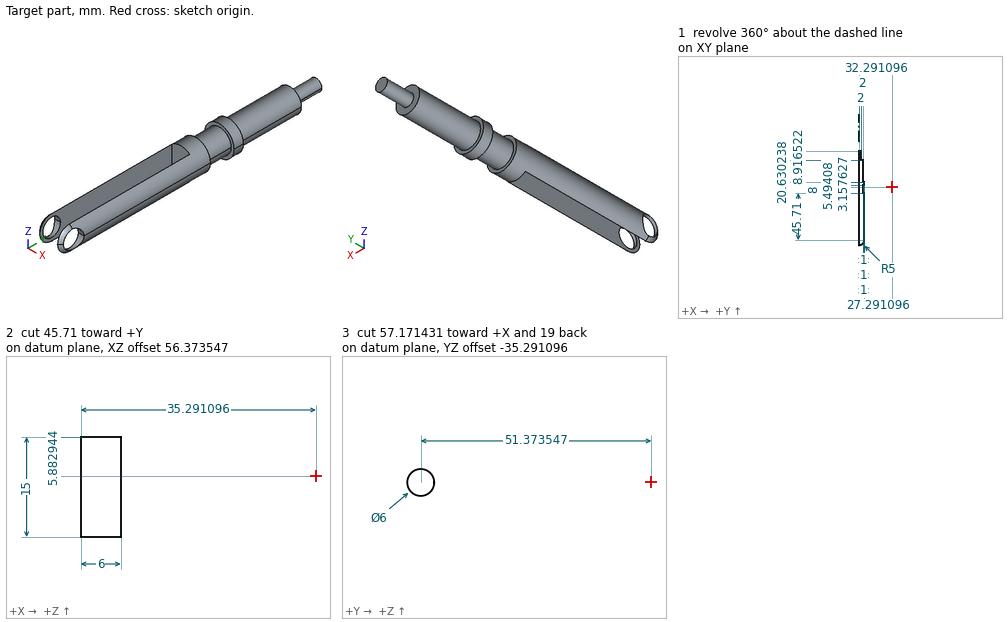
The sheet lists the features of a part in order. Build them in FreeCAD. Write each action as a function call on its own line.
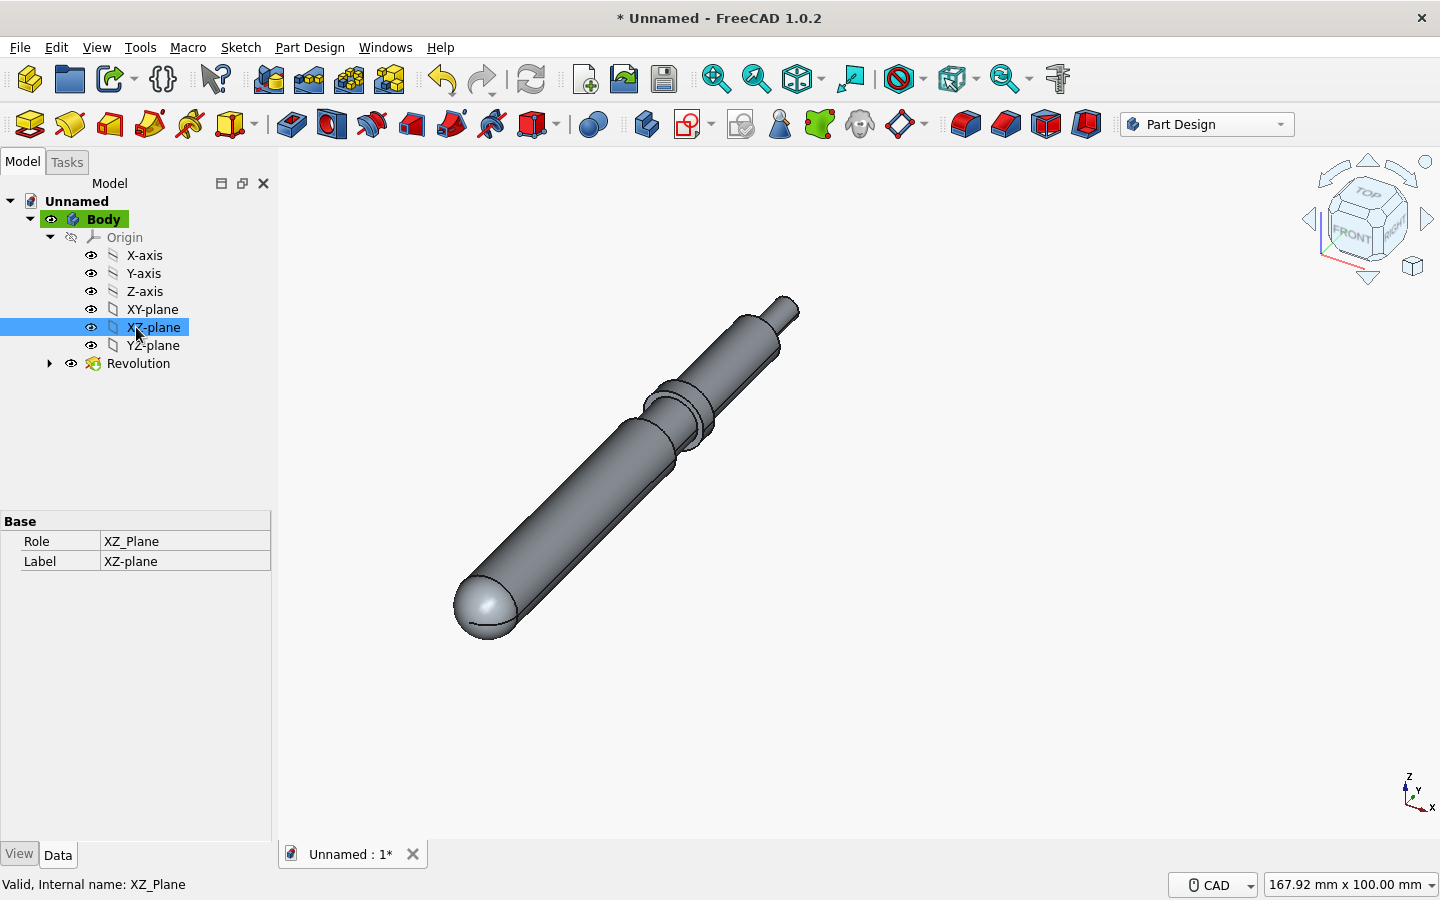
click(900, 124)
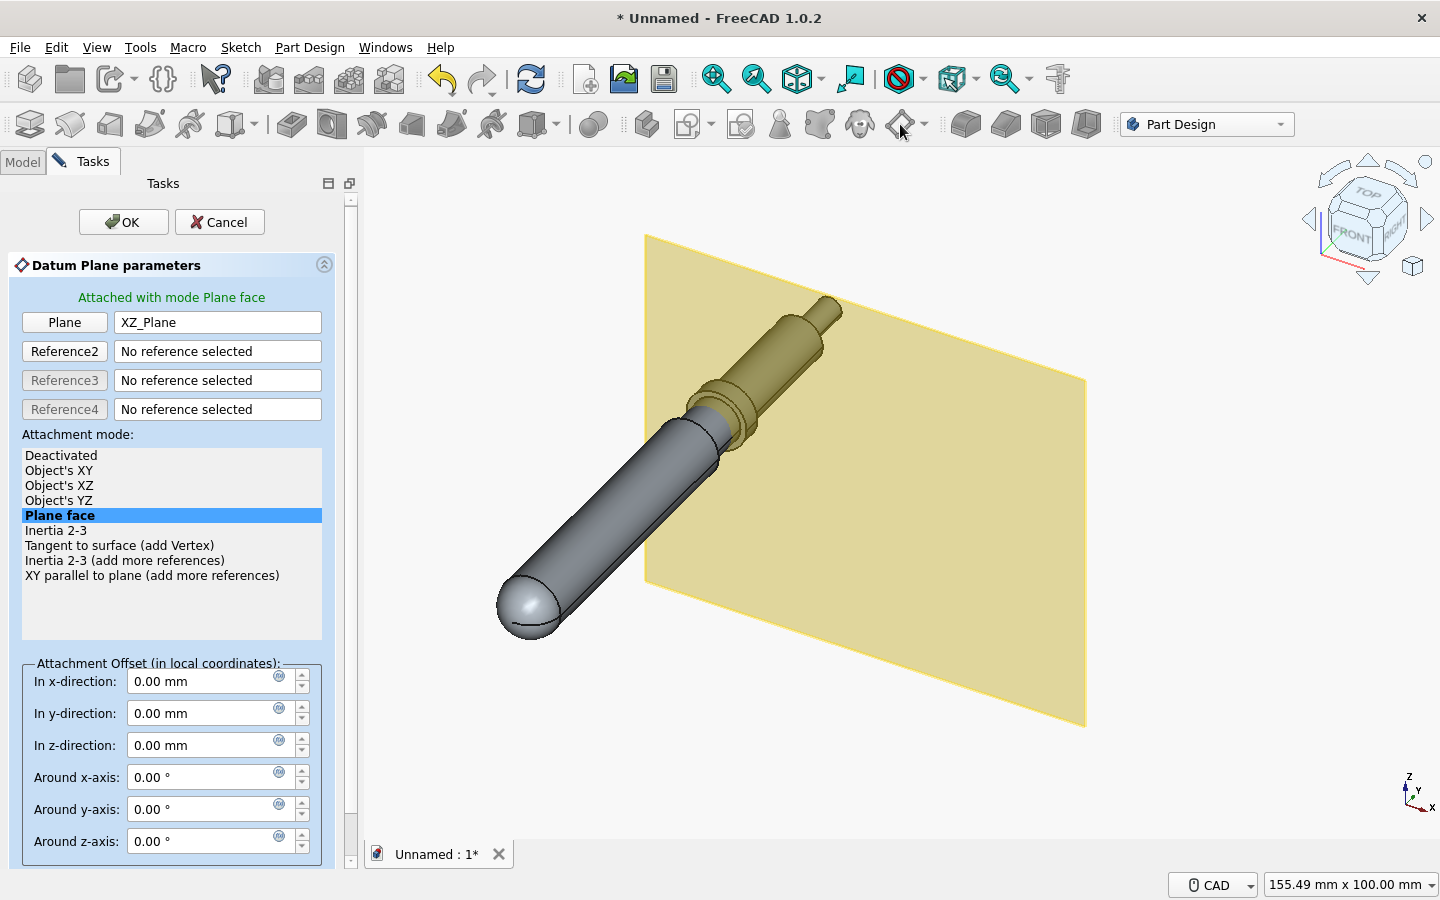
triple_click(210, 745)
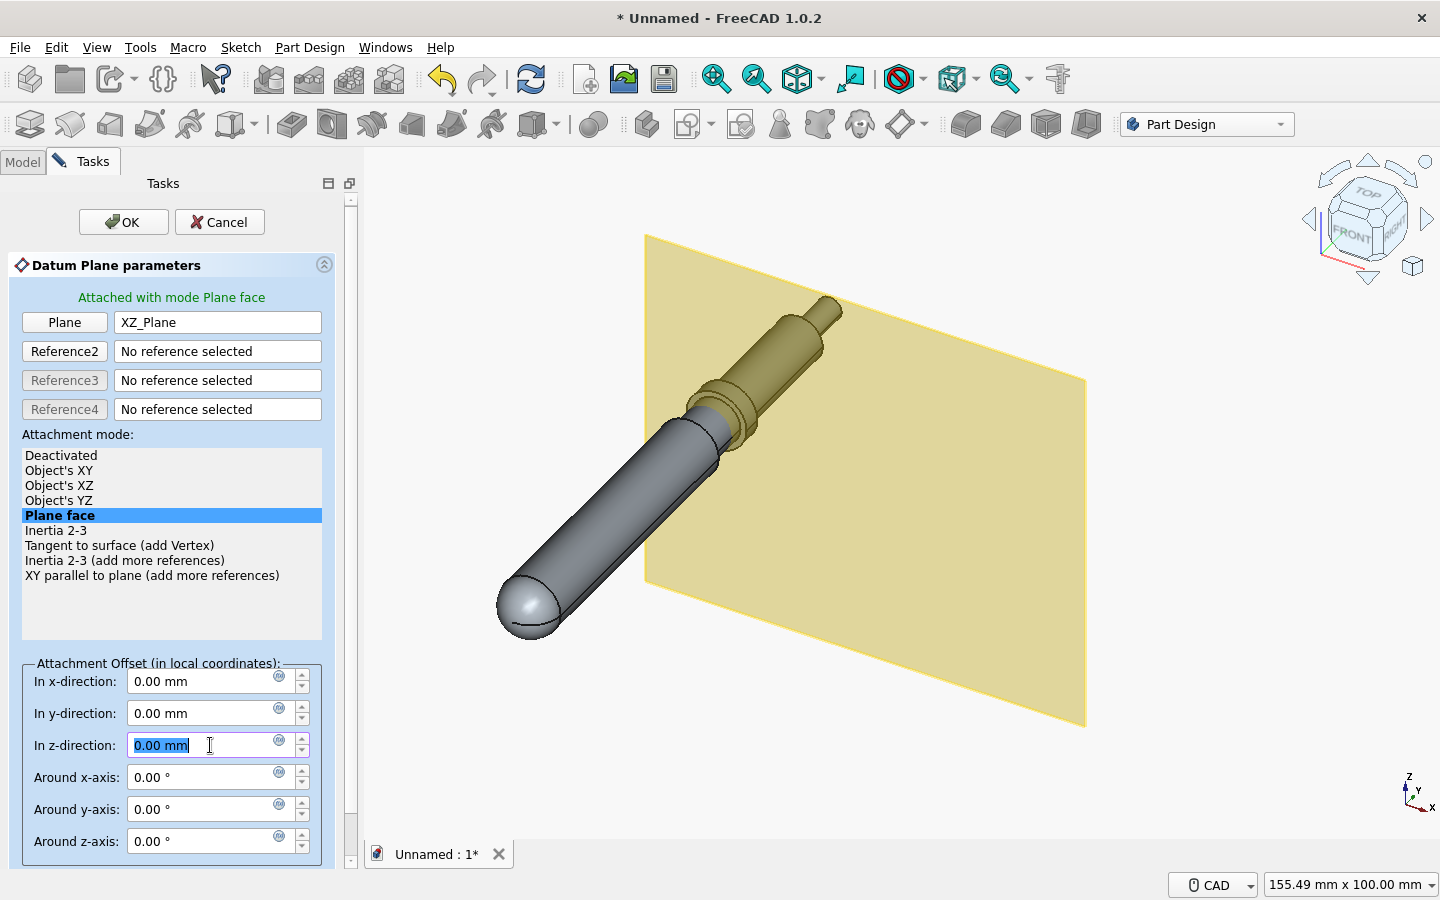
text(56.373547)
key(Tab)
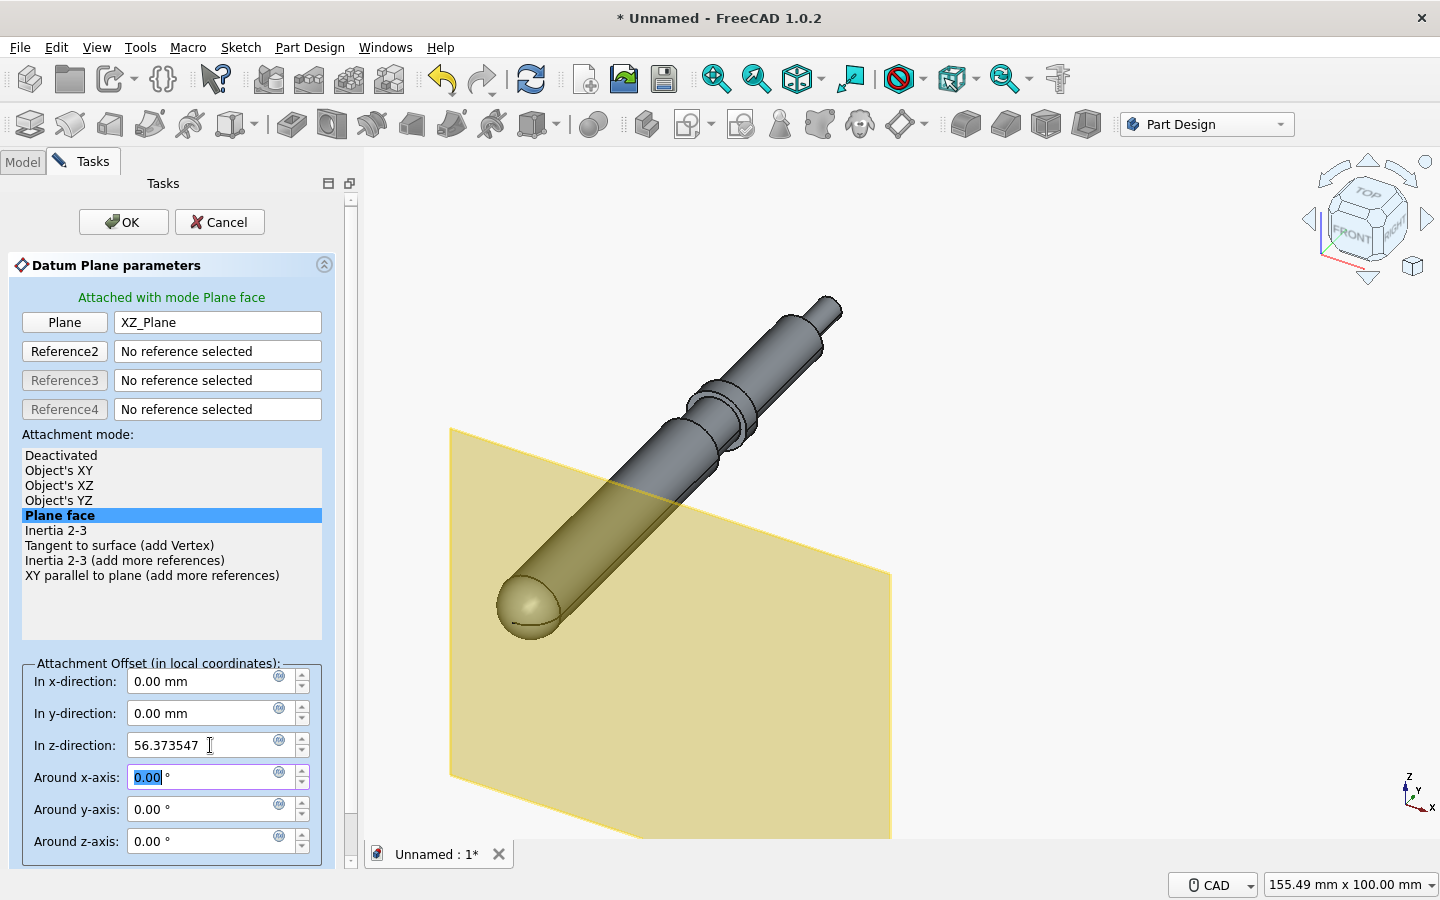
click(124, 222)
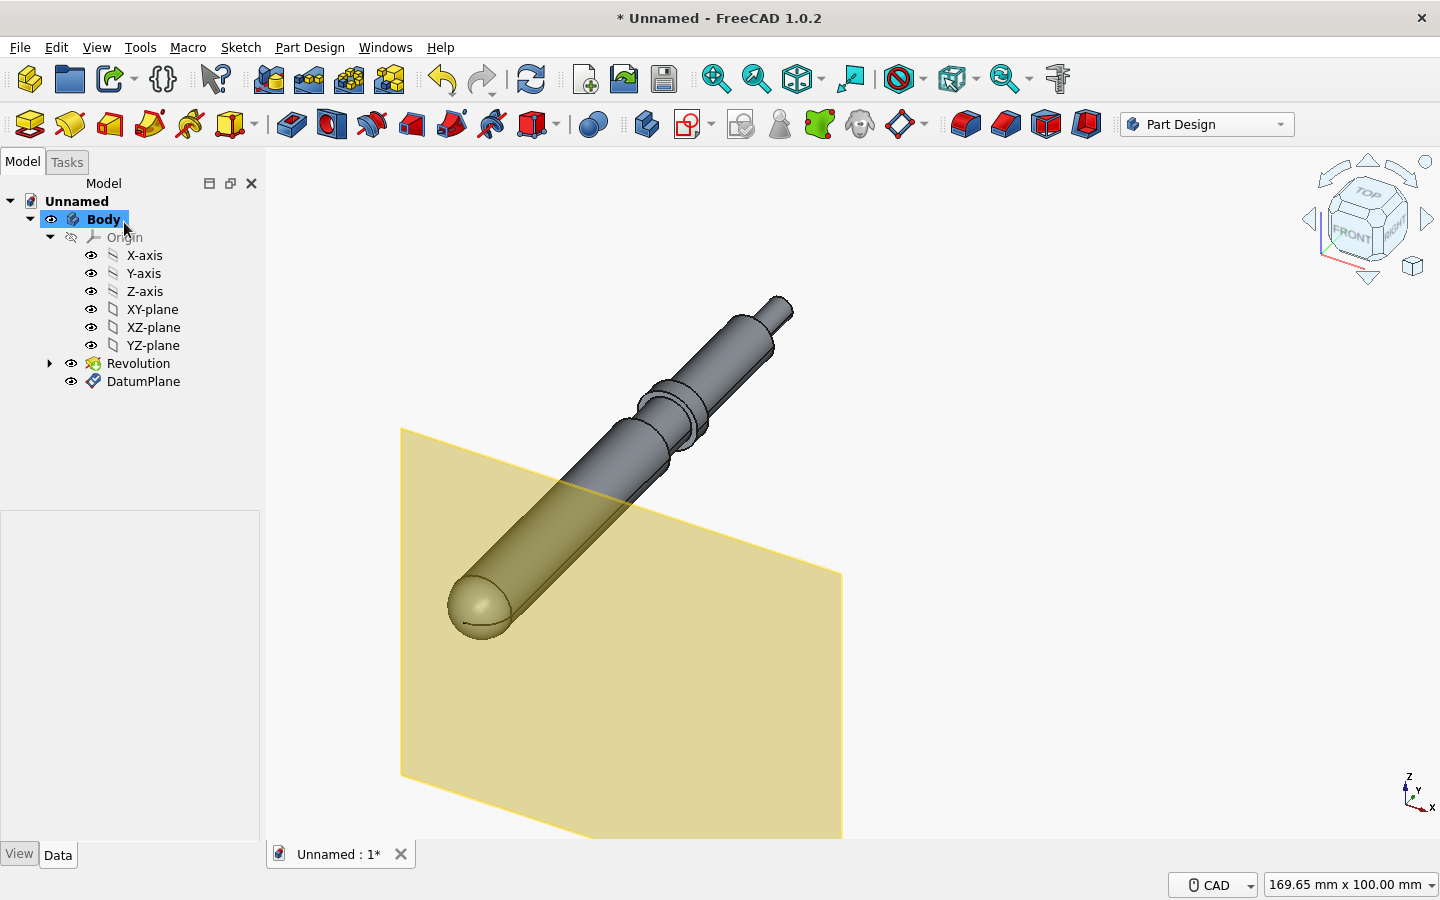
click(116, 381)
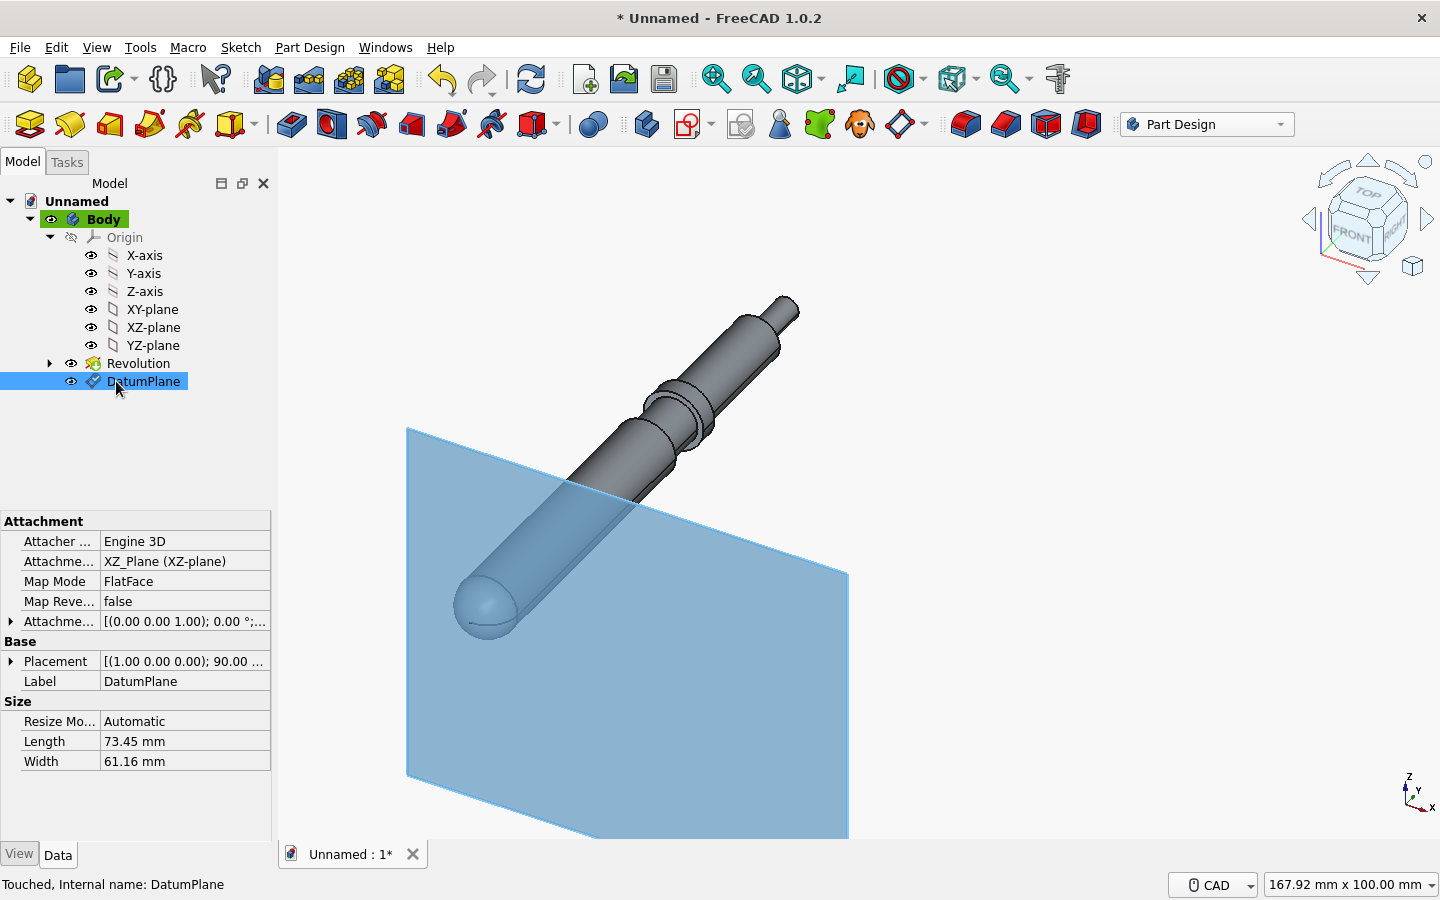
click(688, 124)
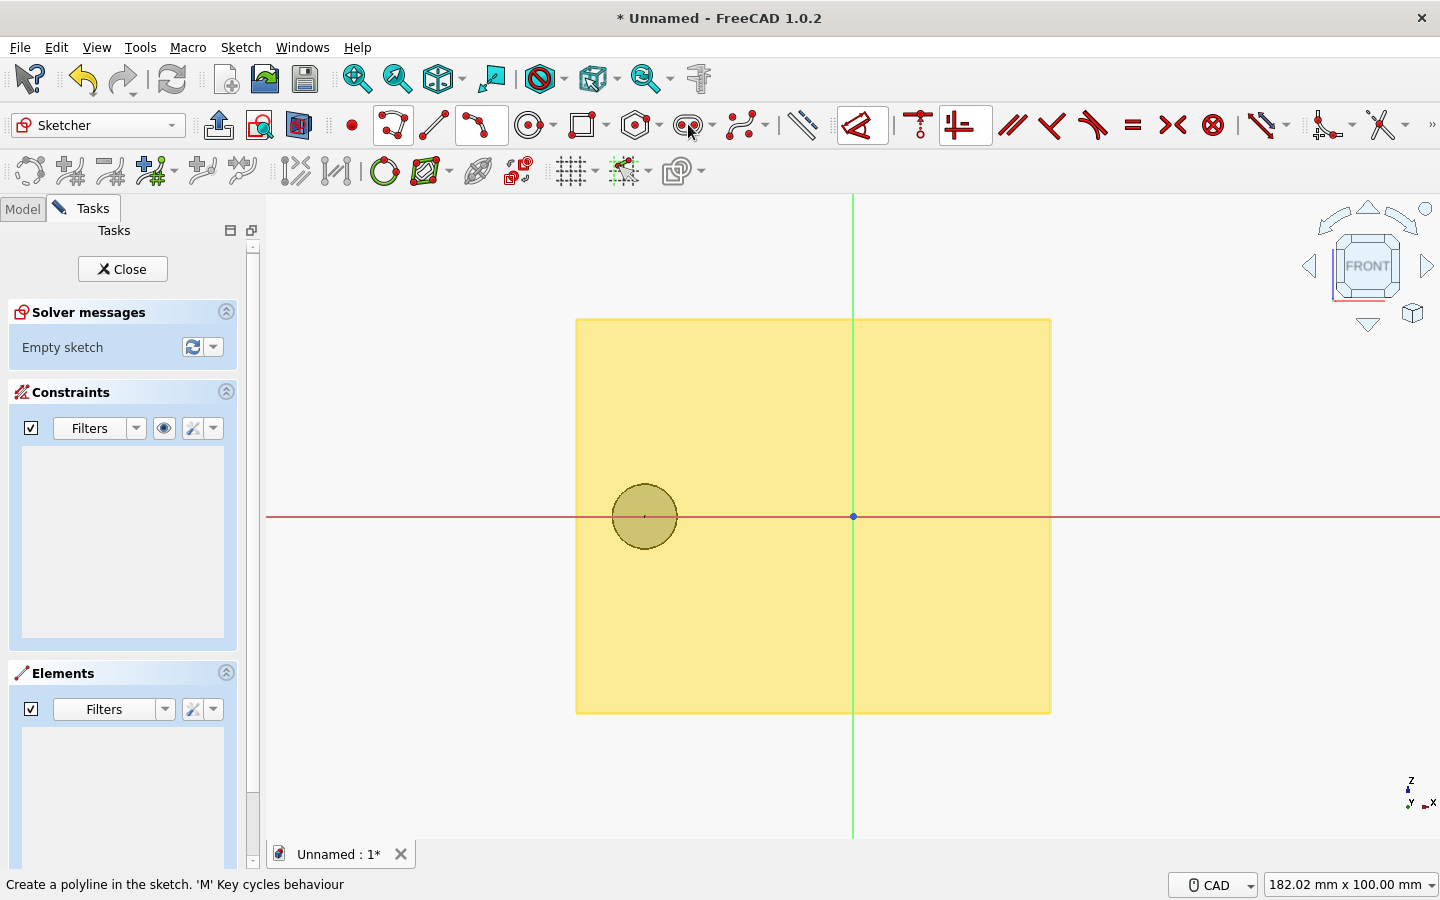
scroll(720, 531, up, 6)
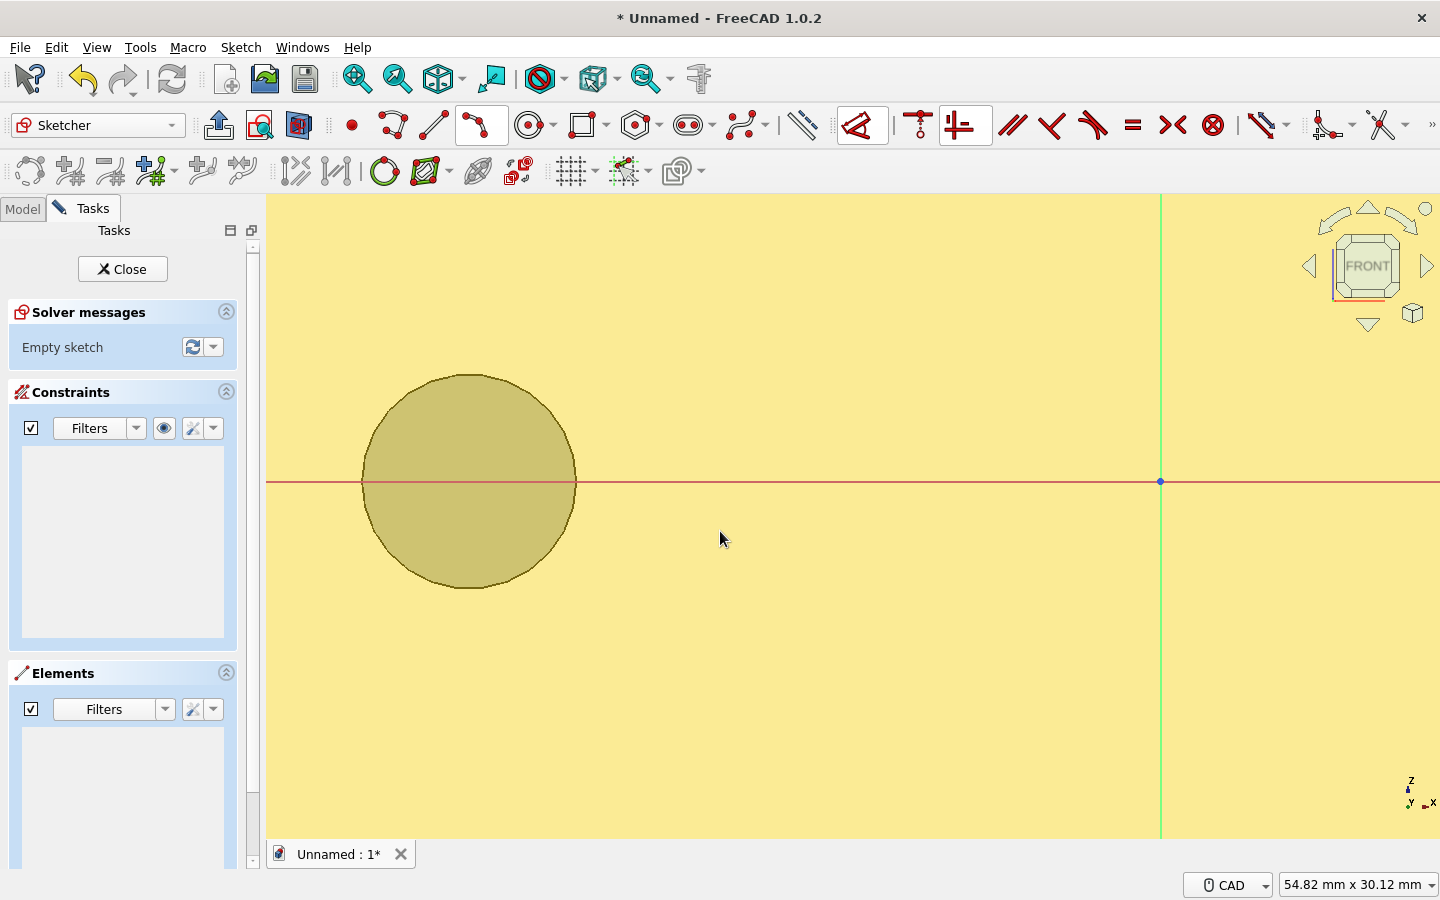
click(582, 126)